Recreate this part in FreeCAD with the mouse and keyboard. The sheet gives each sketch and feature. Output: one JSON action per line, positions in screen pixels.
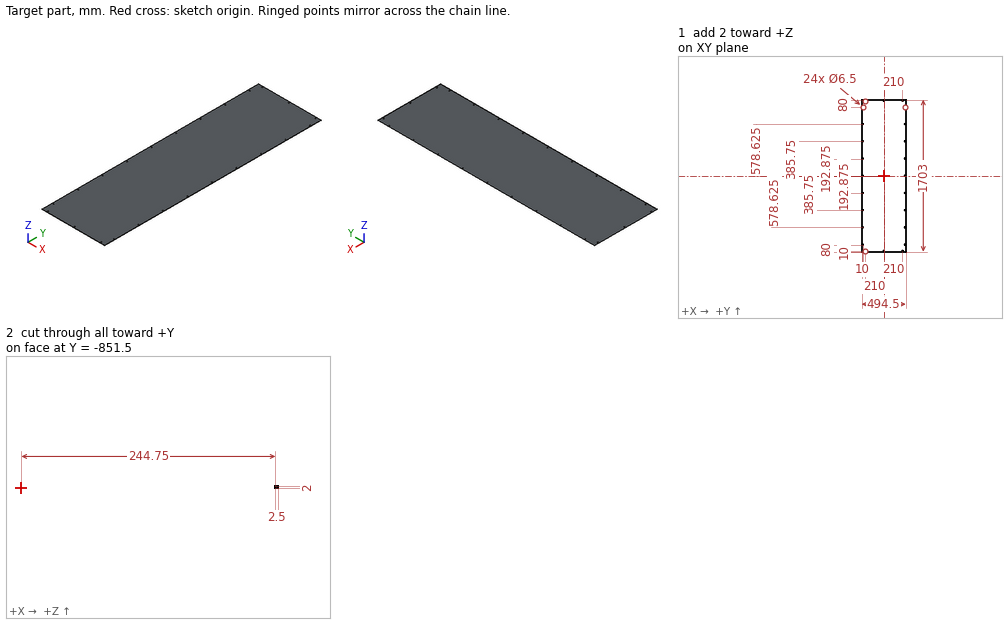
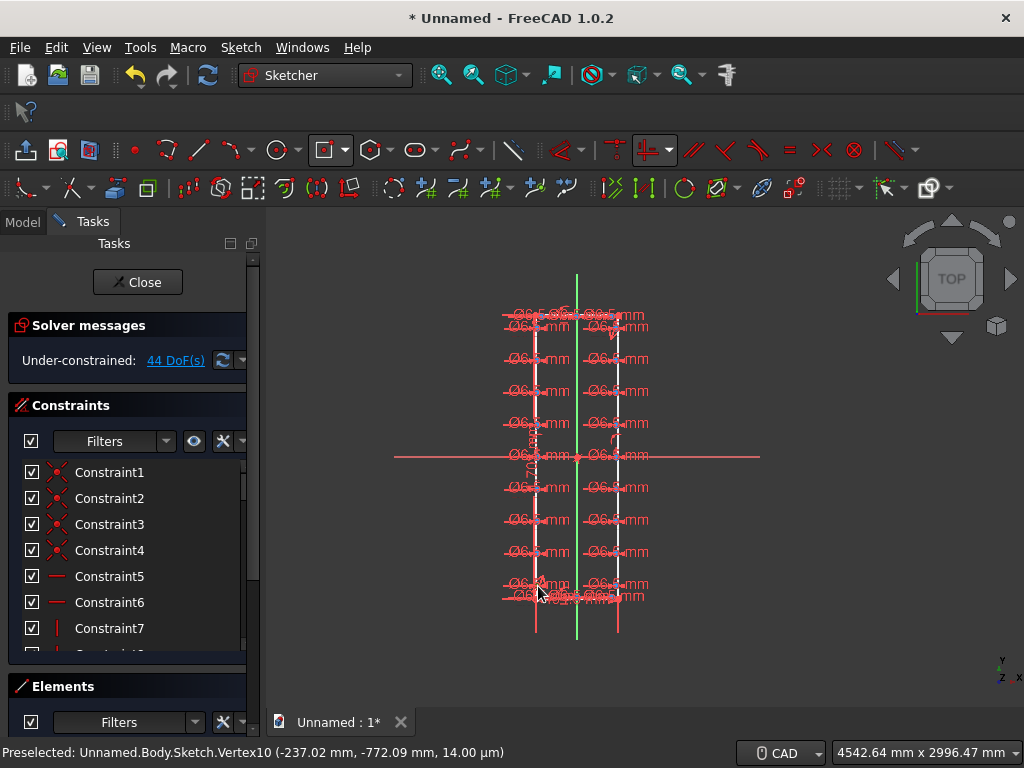
{"action": "left_click", "coordinate": [538, 554]}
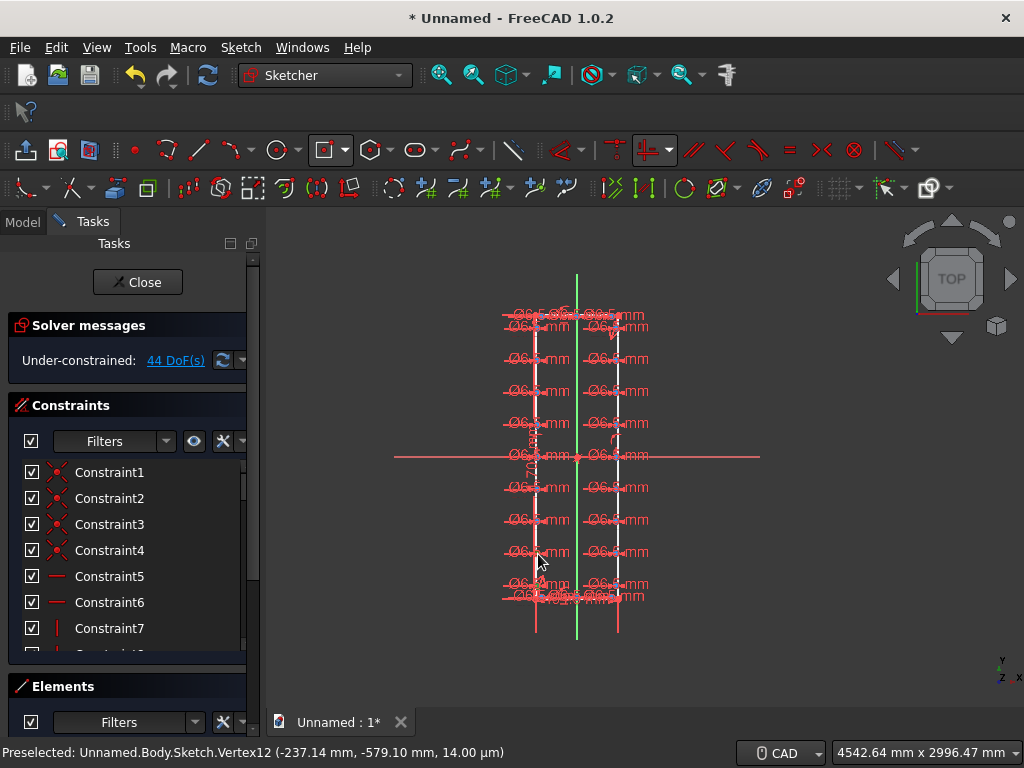
{"action": "left_click", "coordinate": [672, 150]}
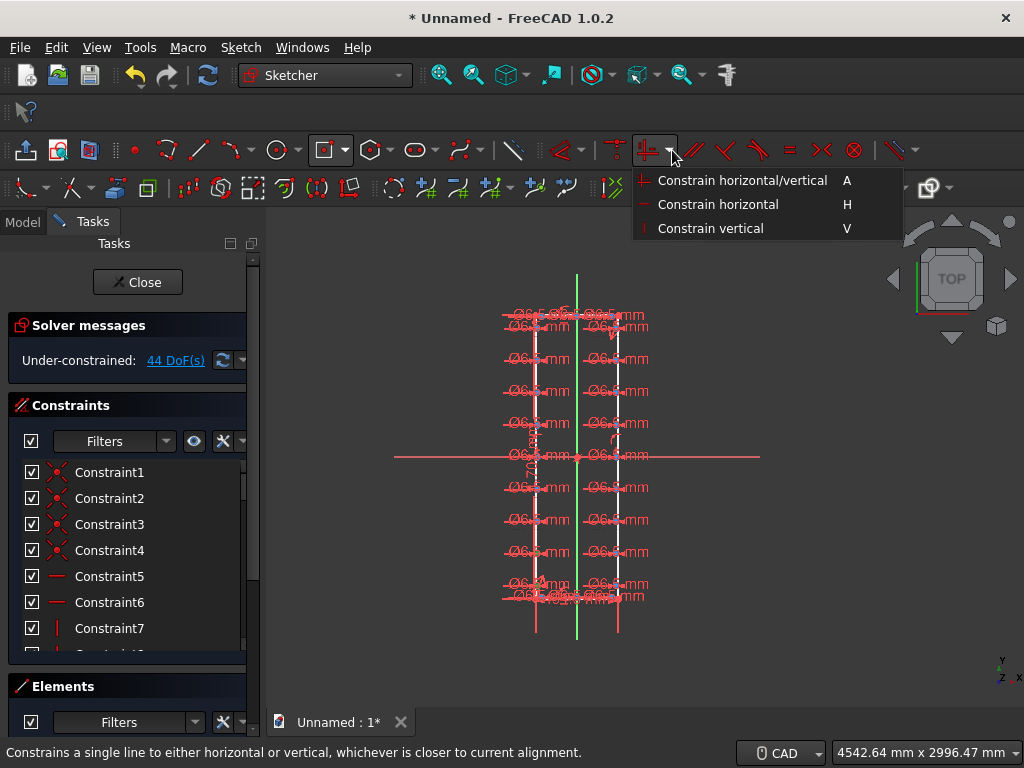
{"action": "left_click", "coordinate": [768, 228]}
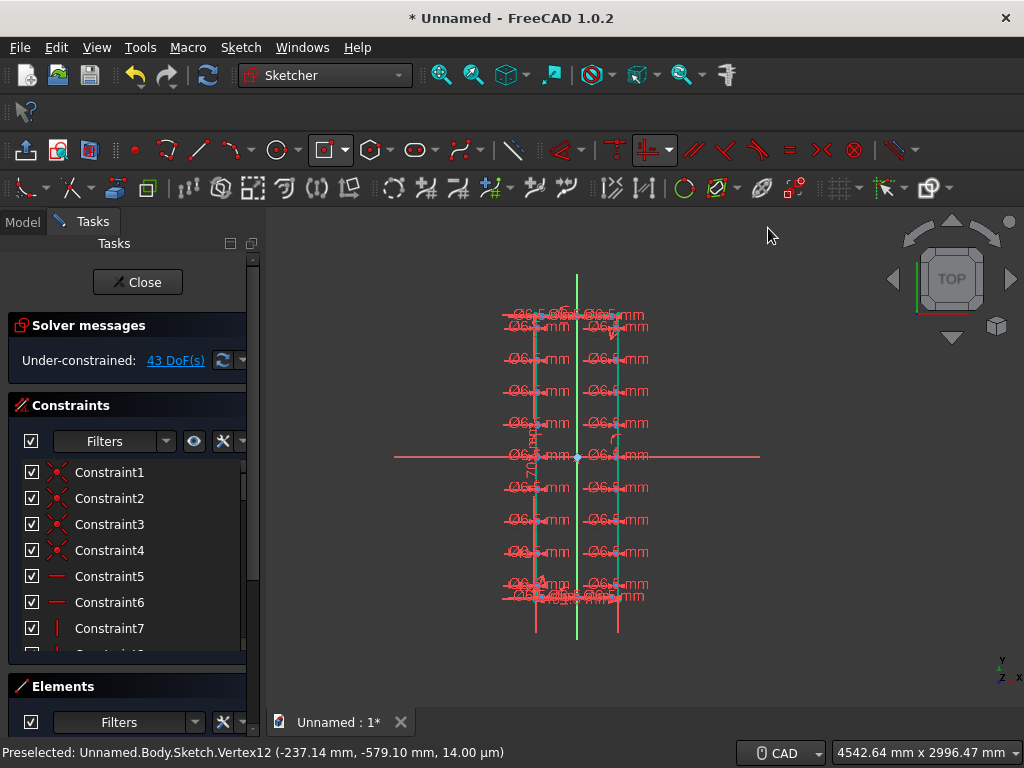
{"action": "left_click", "coordinate": [538, 554]}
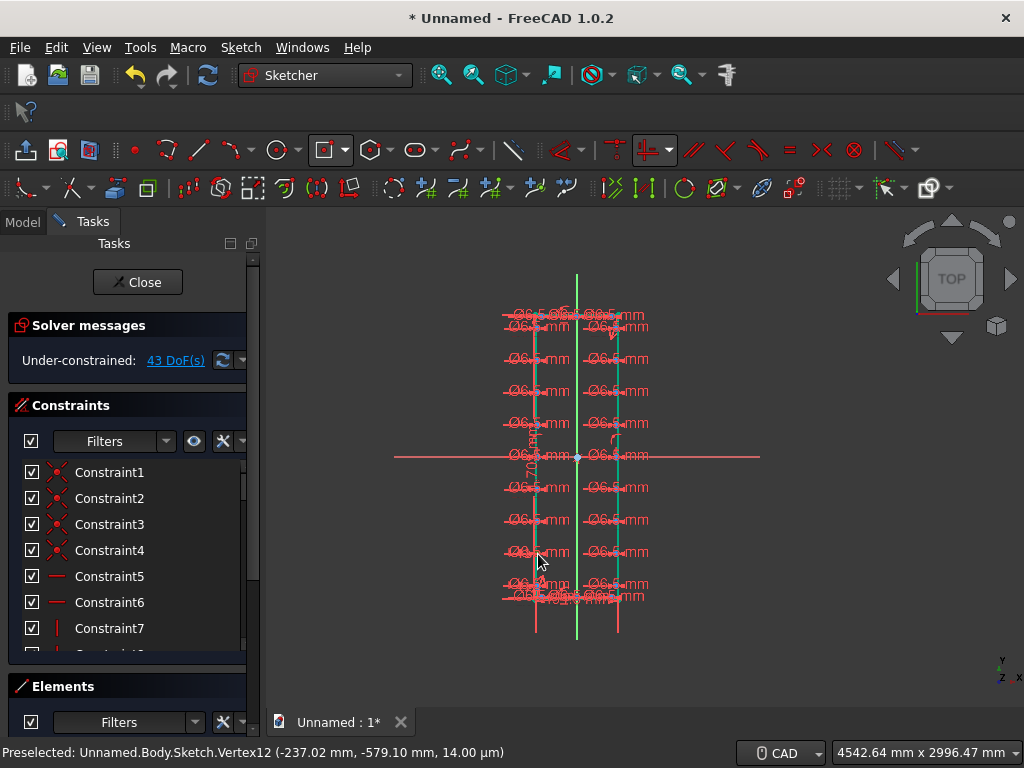
{"action": "left_click", "coordinate": [538, 522]}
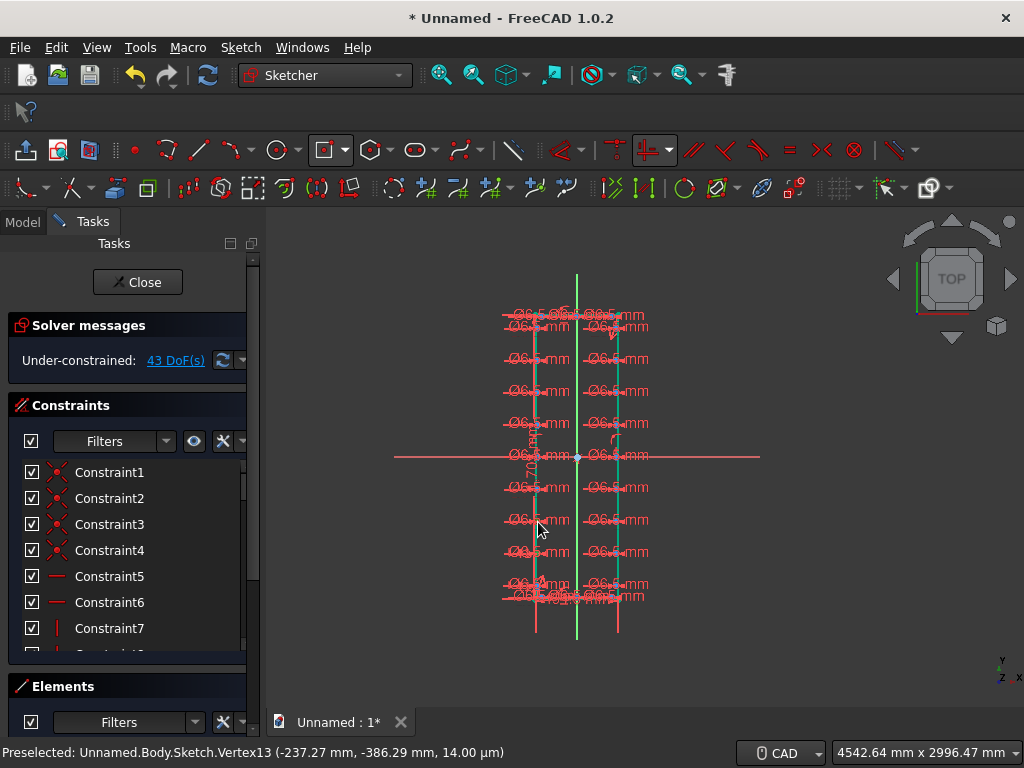
{"action": "key", "text": "v"}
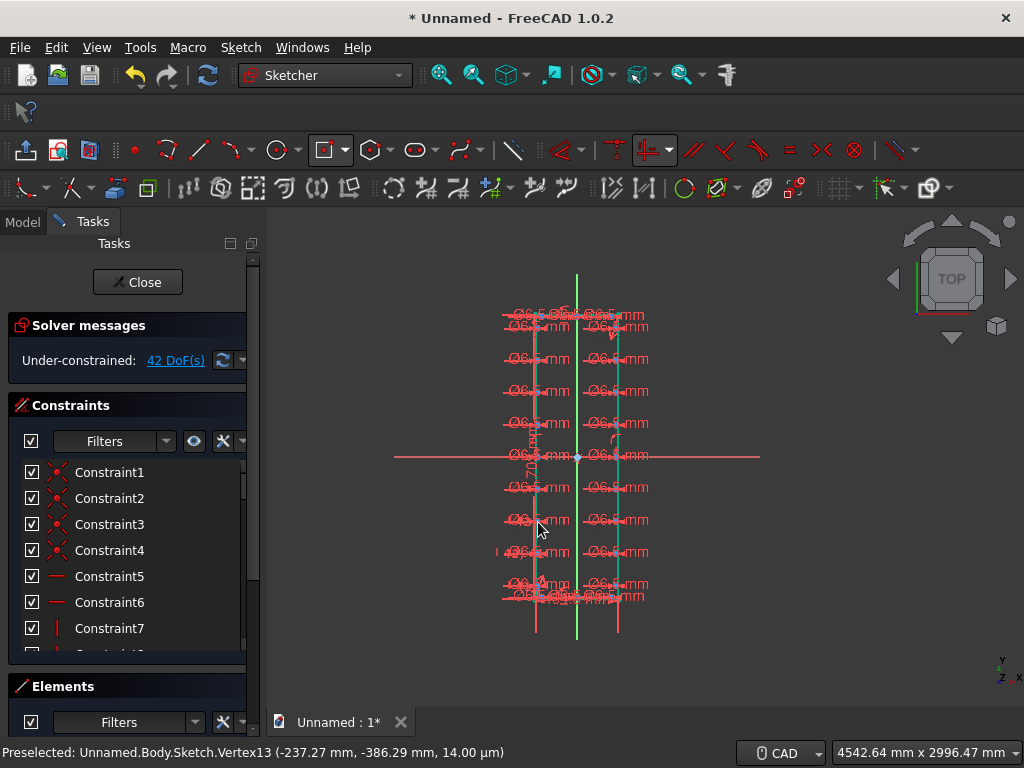
{"action": "left_click", "coordinate": [538, 522]}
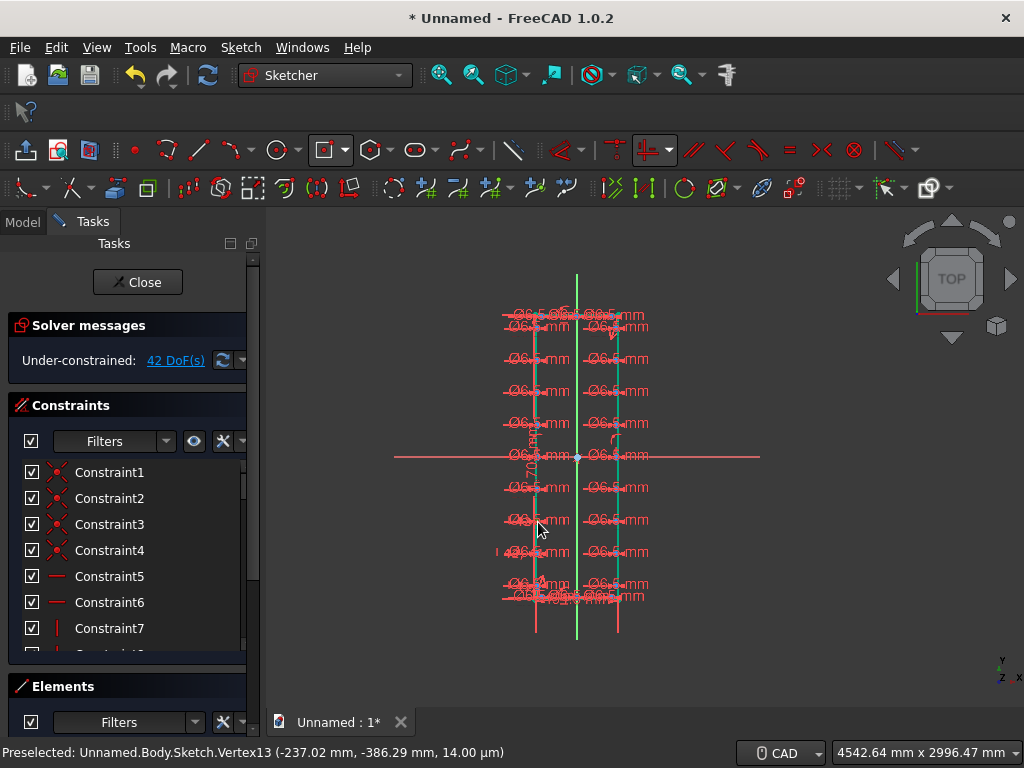
{"action": "left_click", "coordinate": [537, 490]}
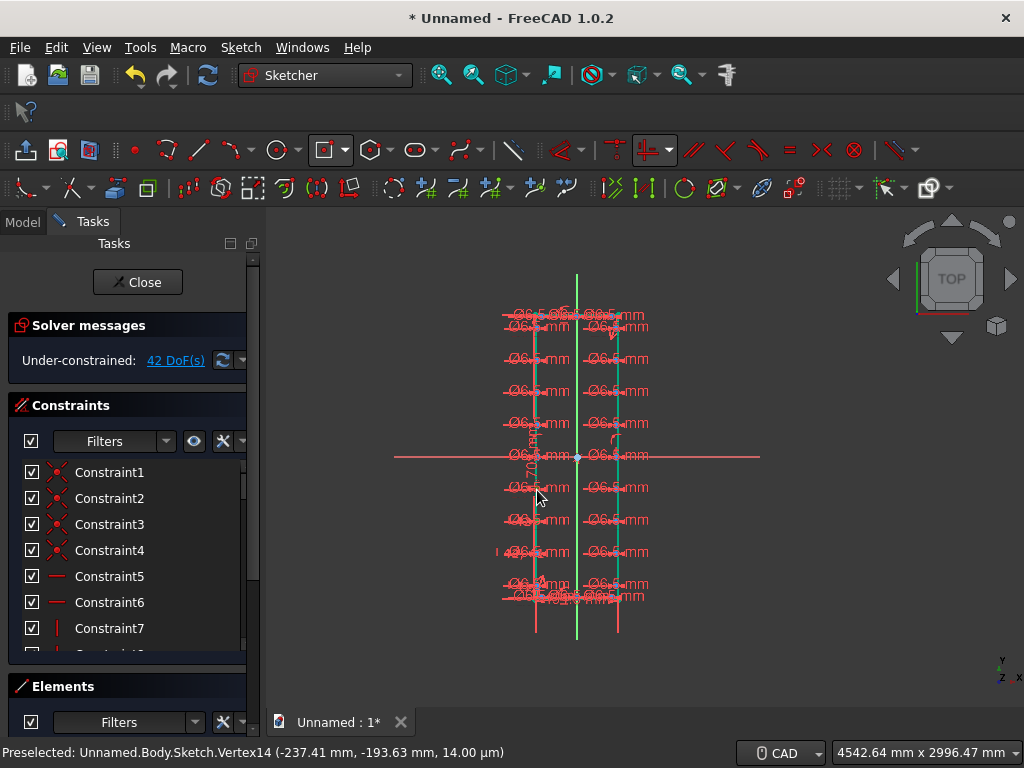
{"action": "left_click", "coordinate": [672, 150]}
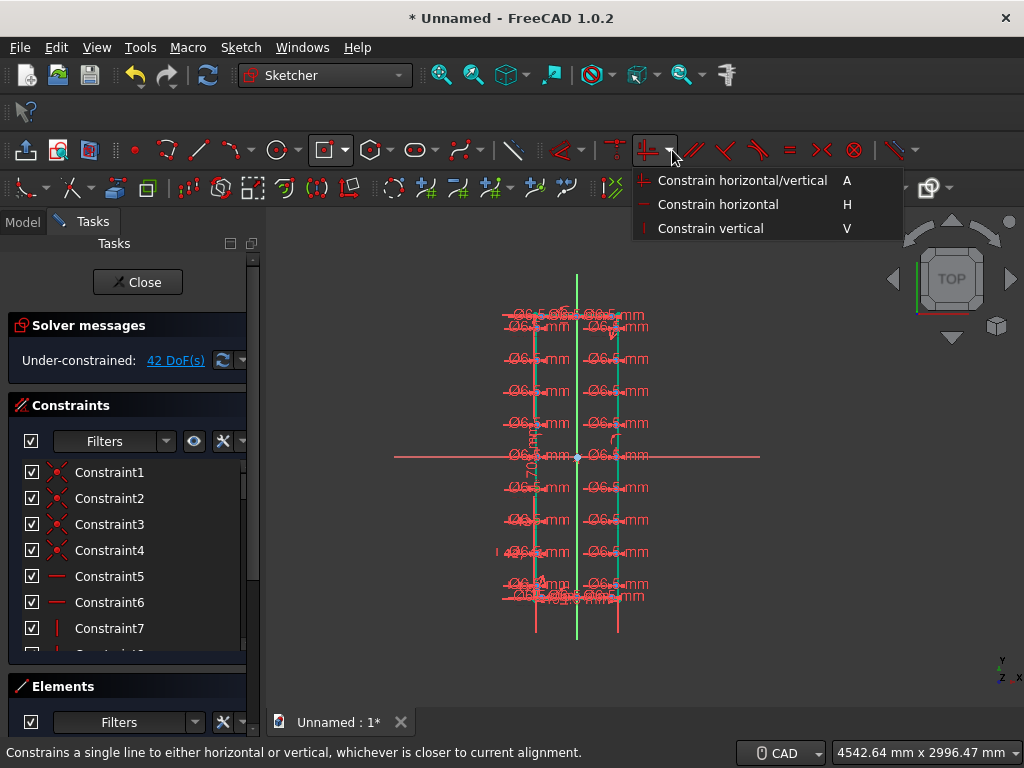
{"action": "left_click", "coordinate": [768, 228]}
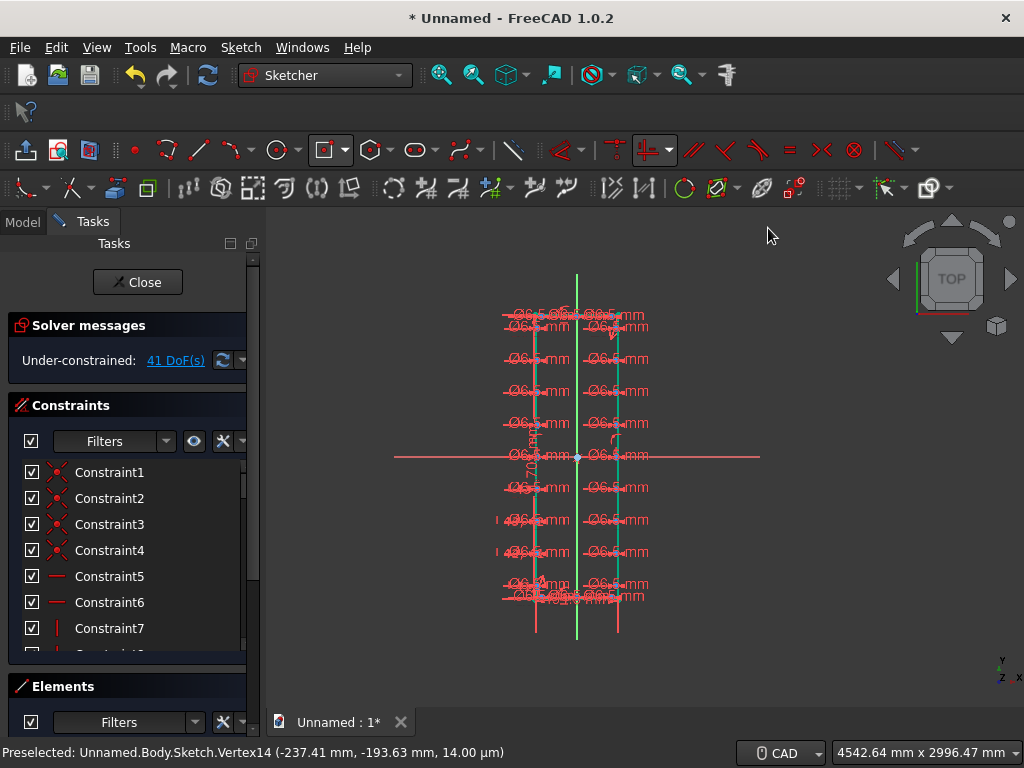
{"action": "scroll", "coordinate": [542, 598], "scroll_direction": "up", "scroll_amount": 4}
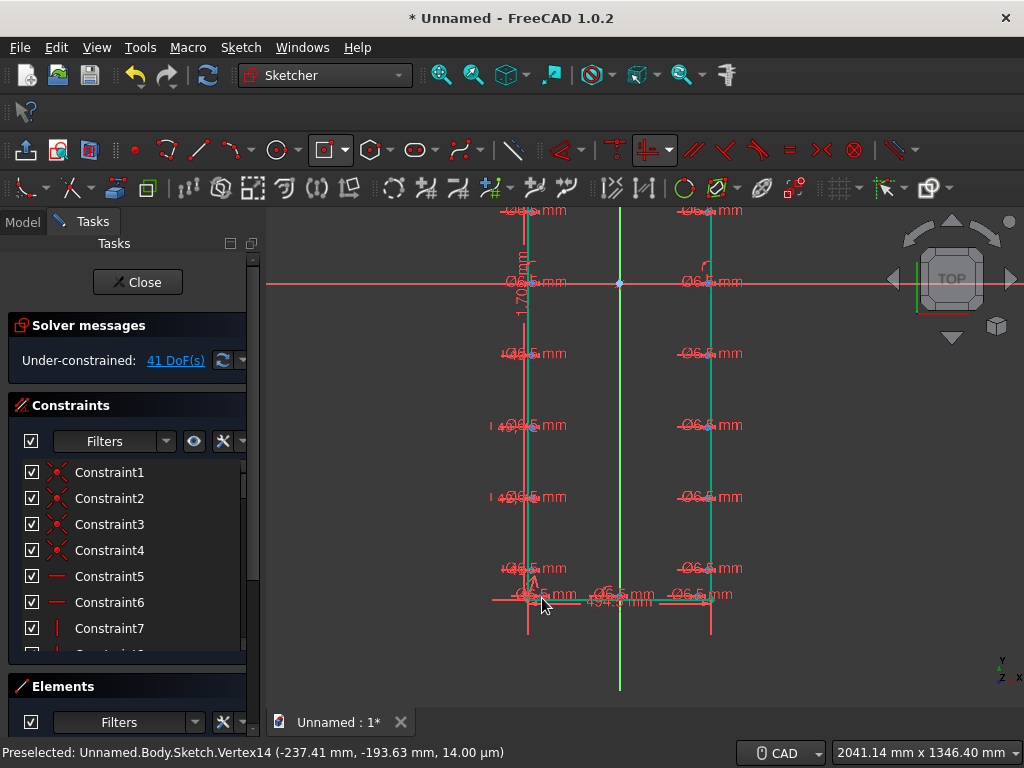
{"action": "left_click", "coordinate": [542, 596]}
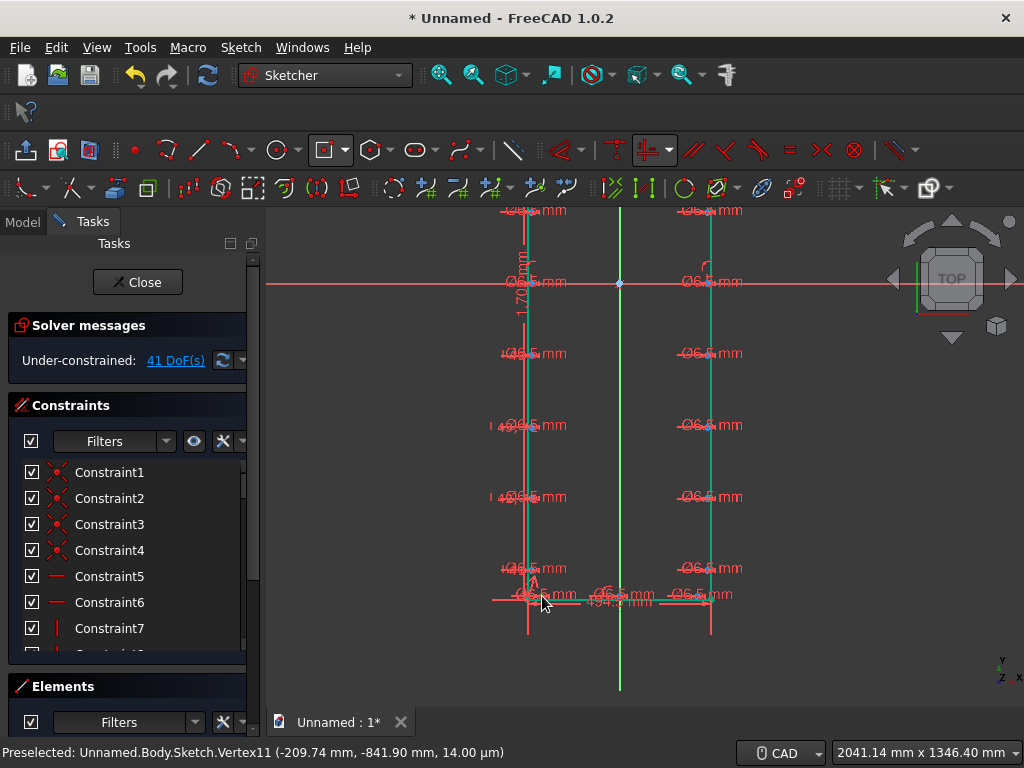
{"action": "left_click", "coordinate": [620, 596]}